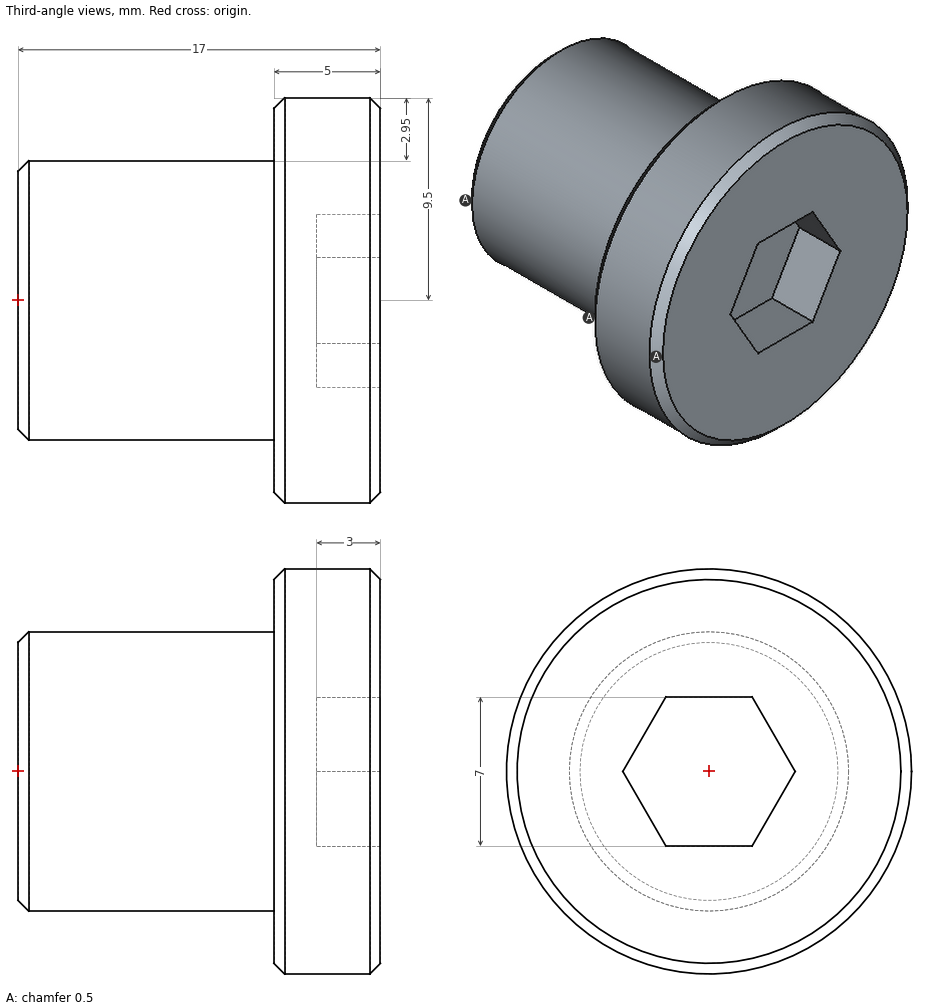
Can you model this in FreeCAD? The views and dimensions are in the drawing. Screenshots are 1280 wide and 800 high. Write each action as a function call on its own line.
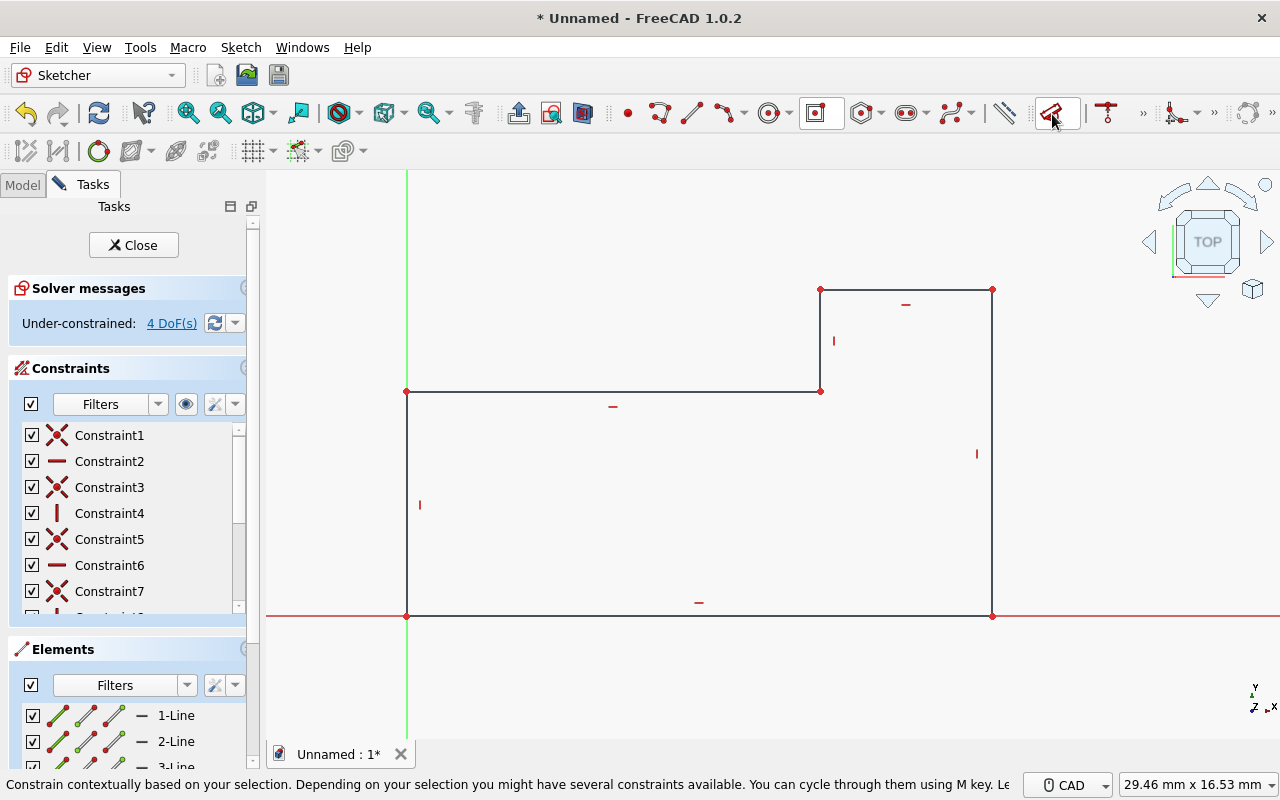
click(940, 290)
click(906, 256)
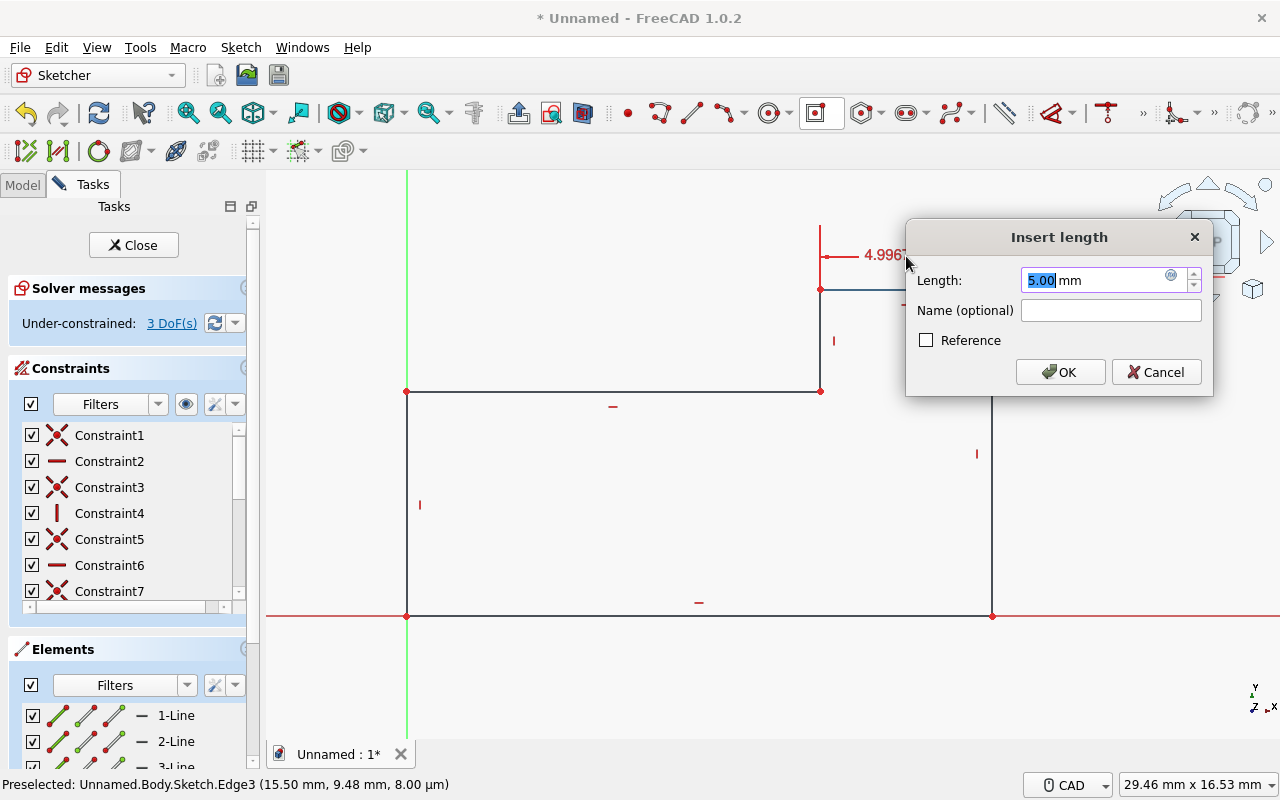
text(5)
key(Return)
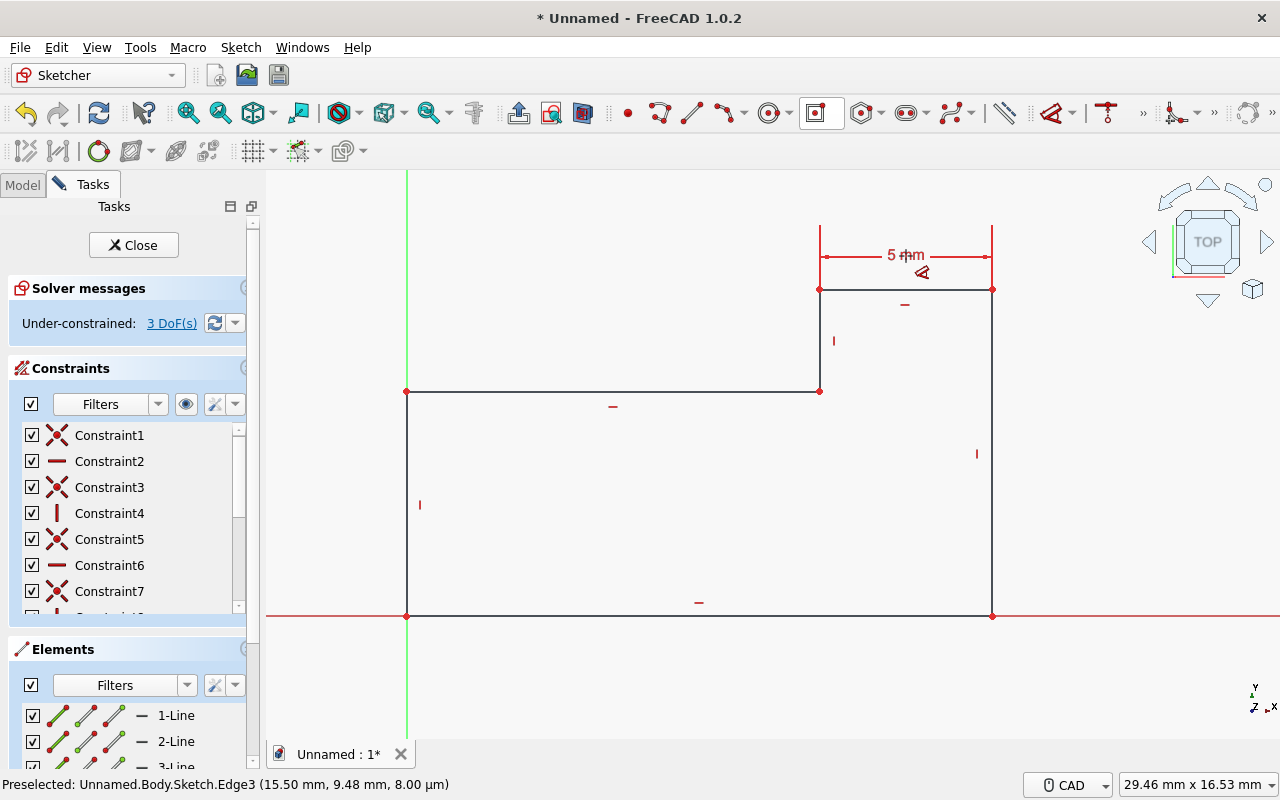
click(582, 616)
click(699, 650)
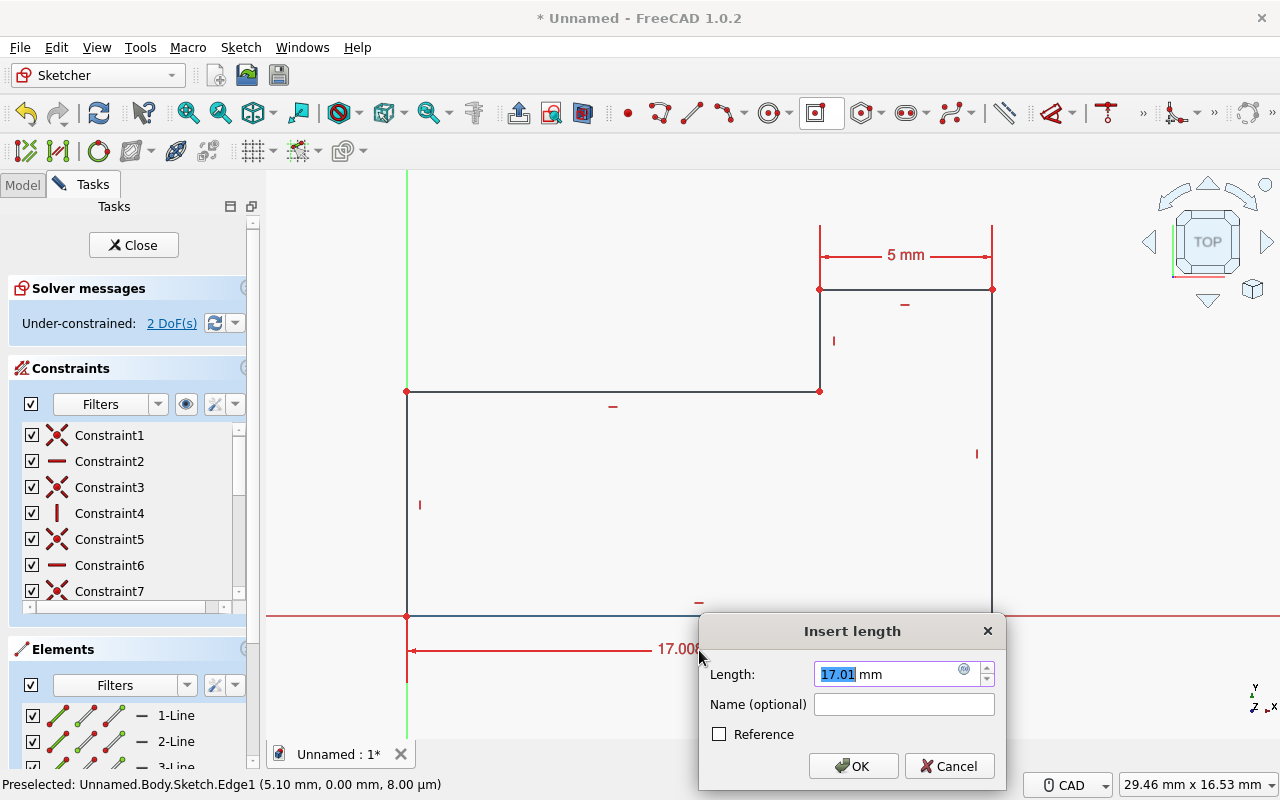
text(17)
key(Return)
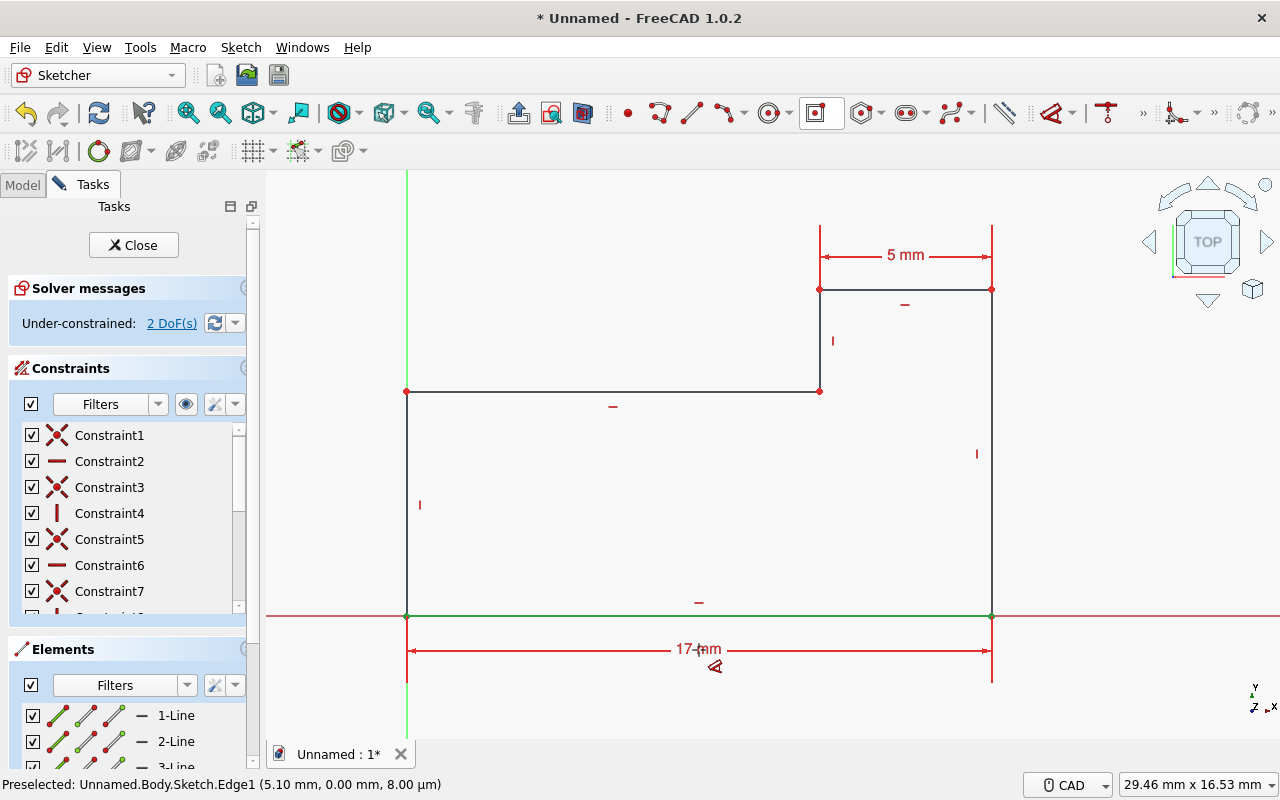
click(992, 518)
click(1026, 453)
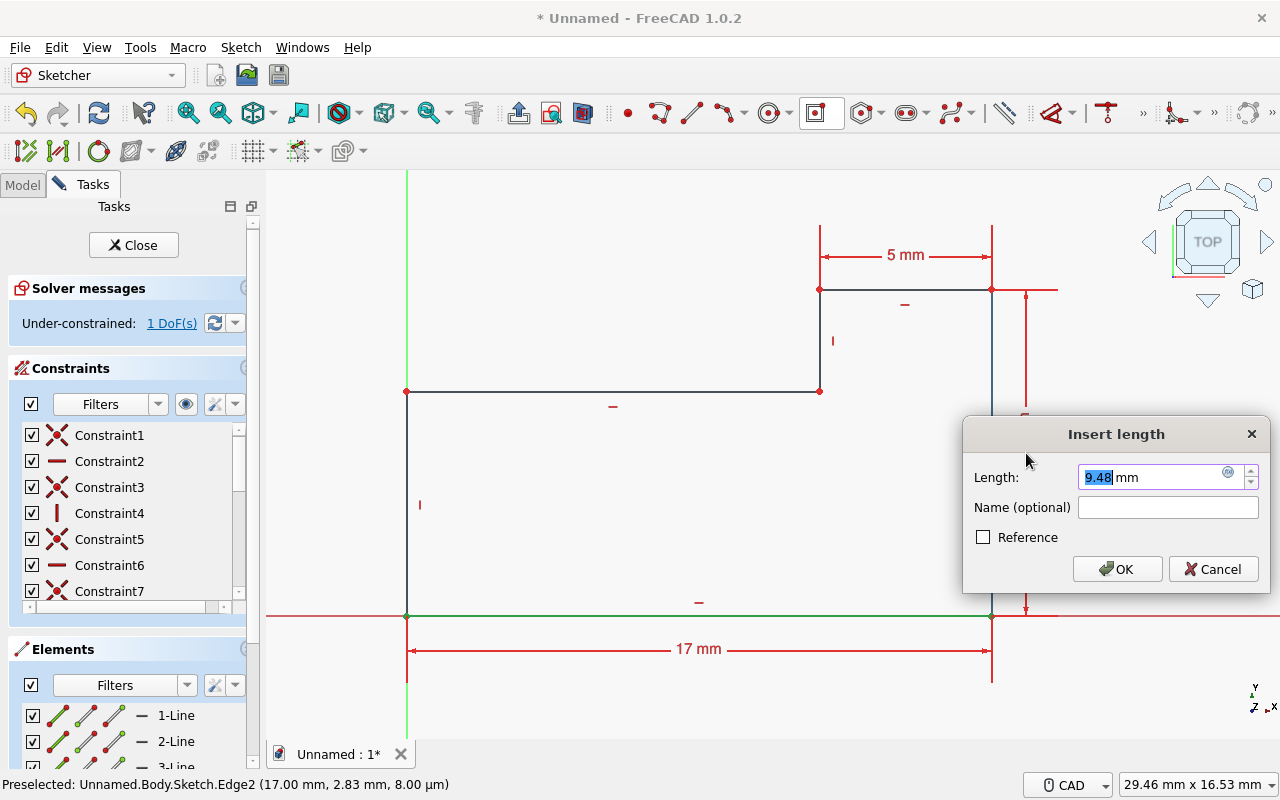
text(9.5)
key(Return)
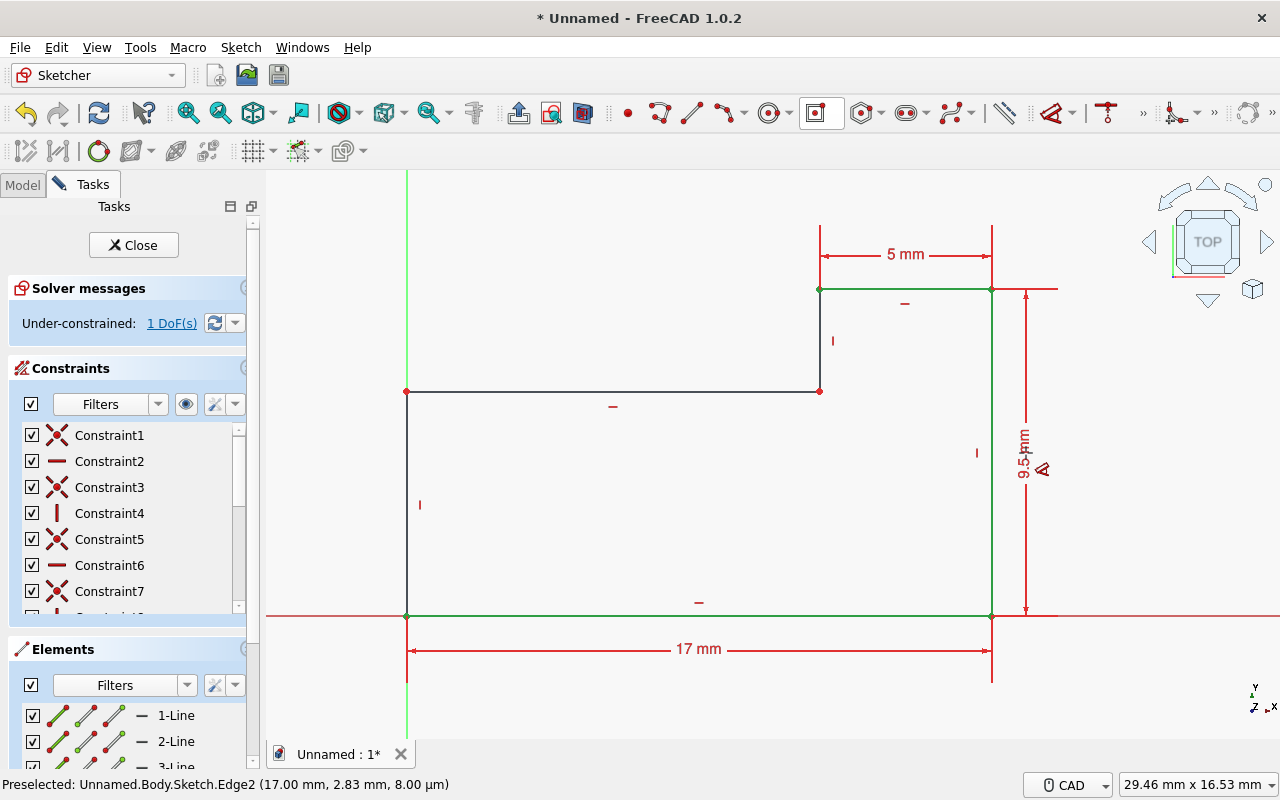
click(820, 320)
click(854, 341)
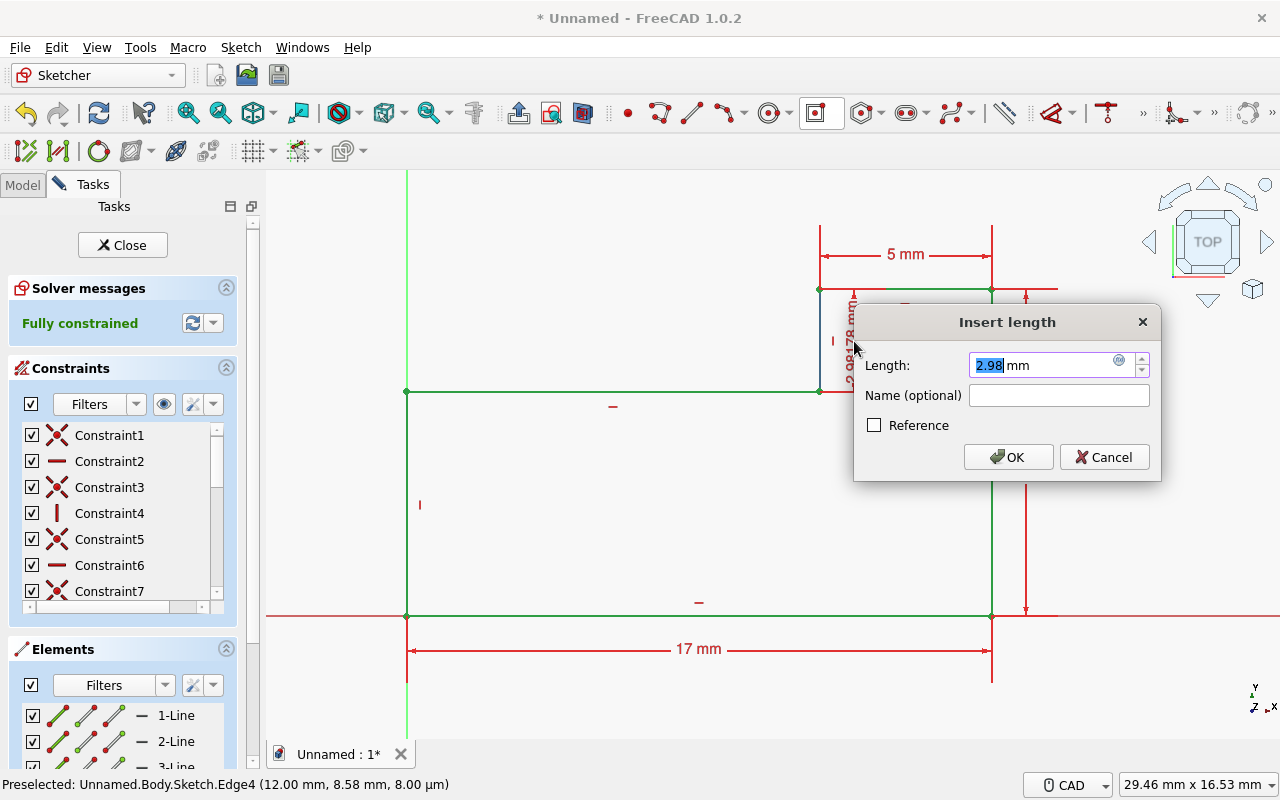
text(2.95)
key(Return)
key(Escape)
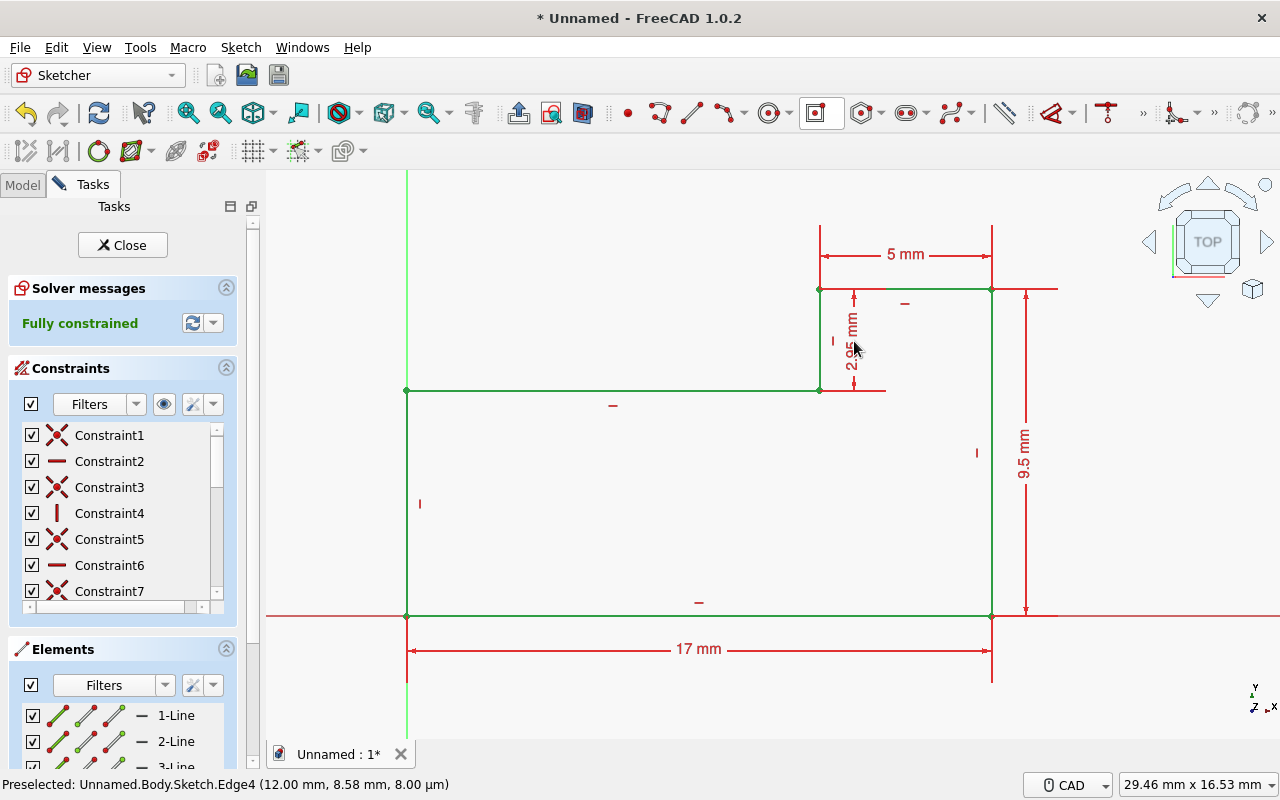
click(123, 245)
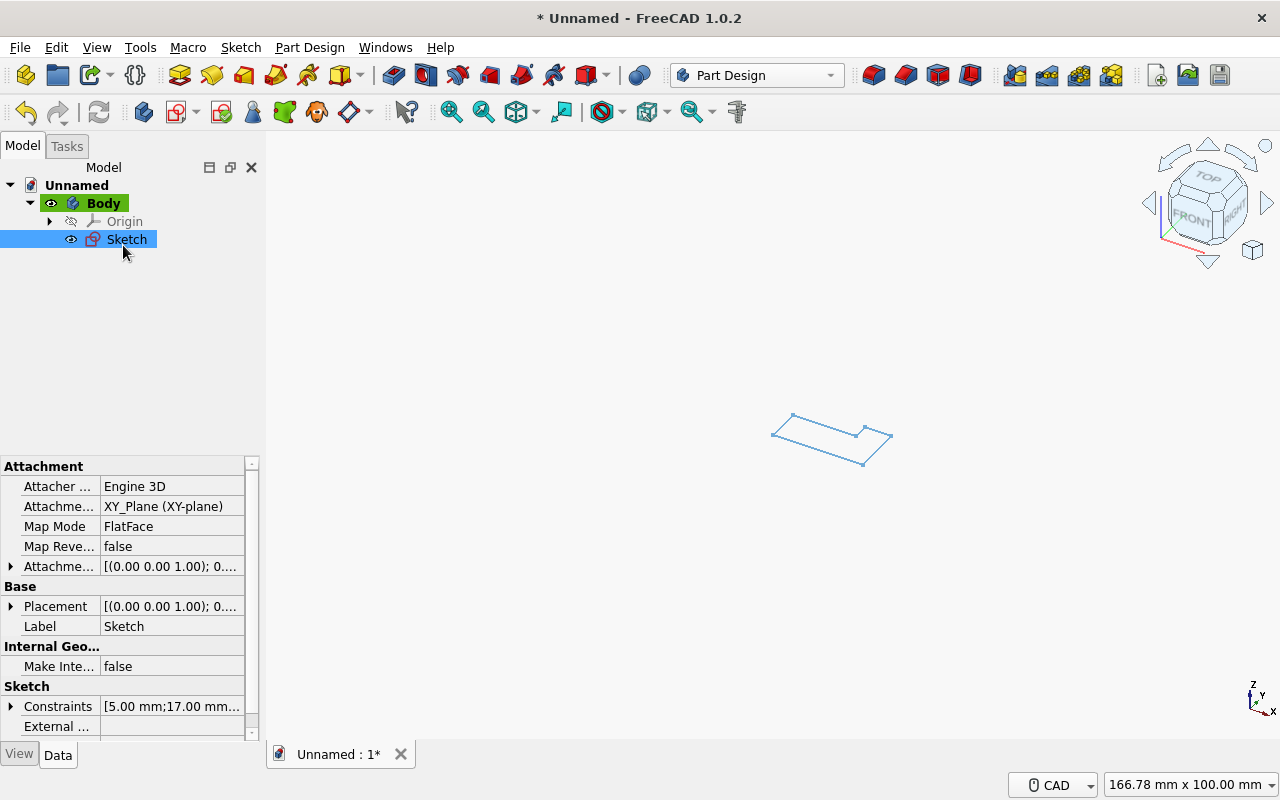
click(212, 76)